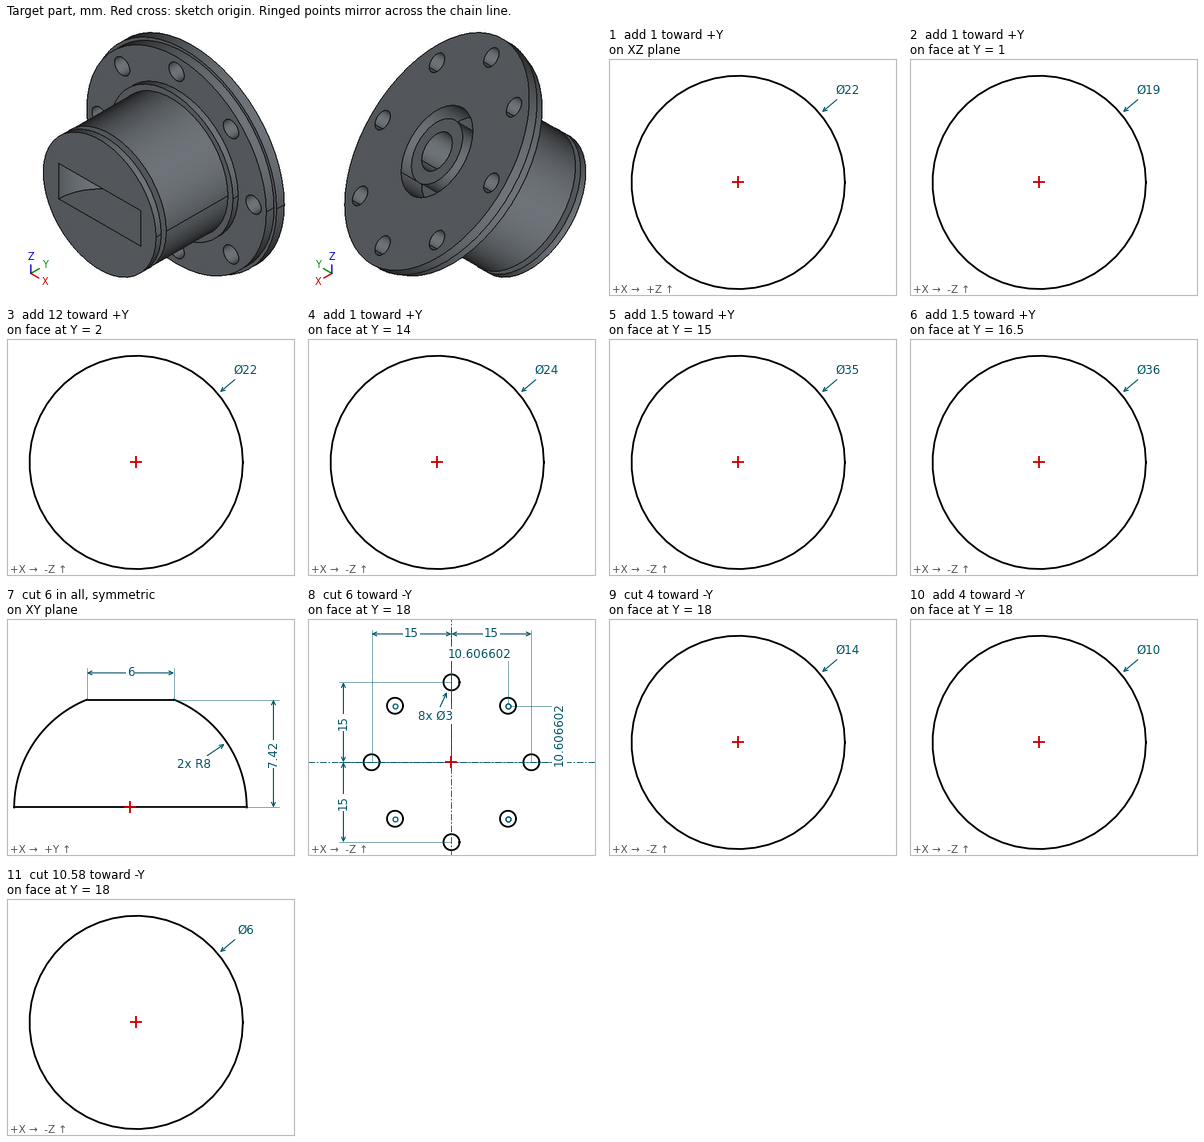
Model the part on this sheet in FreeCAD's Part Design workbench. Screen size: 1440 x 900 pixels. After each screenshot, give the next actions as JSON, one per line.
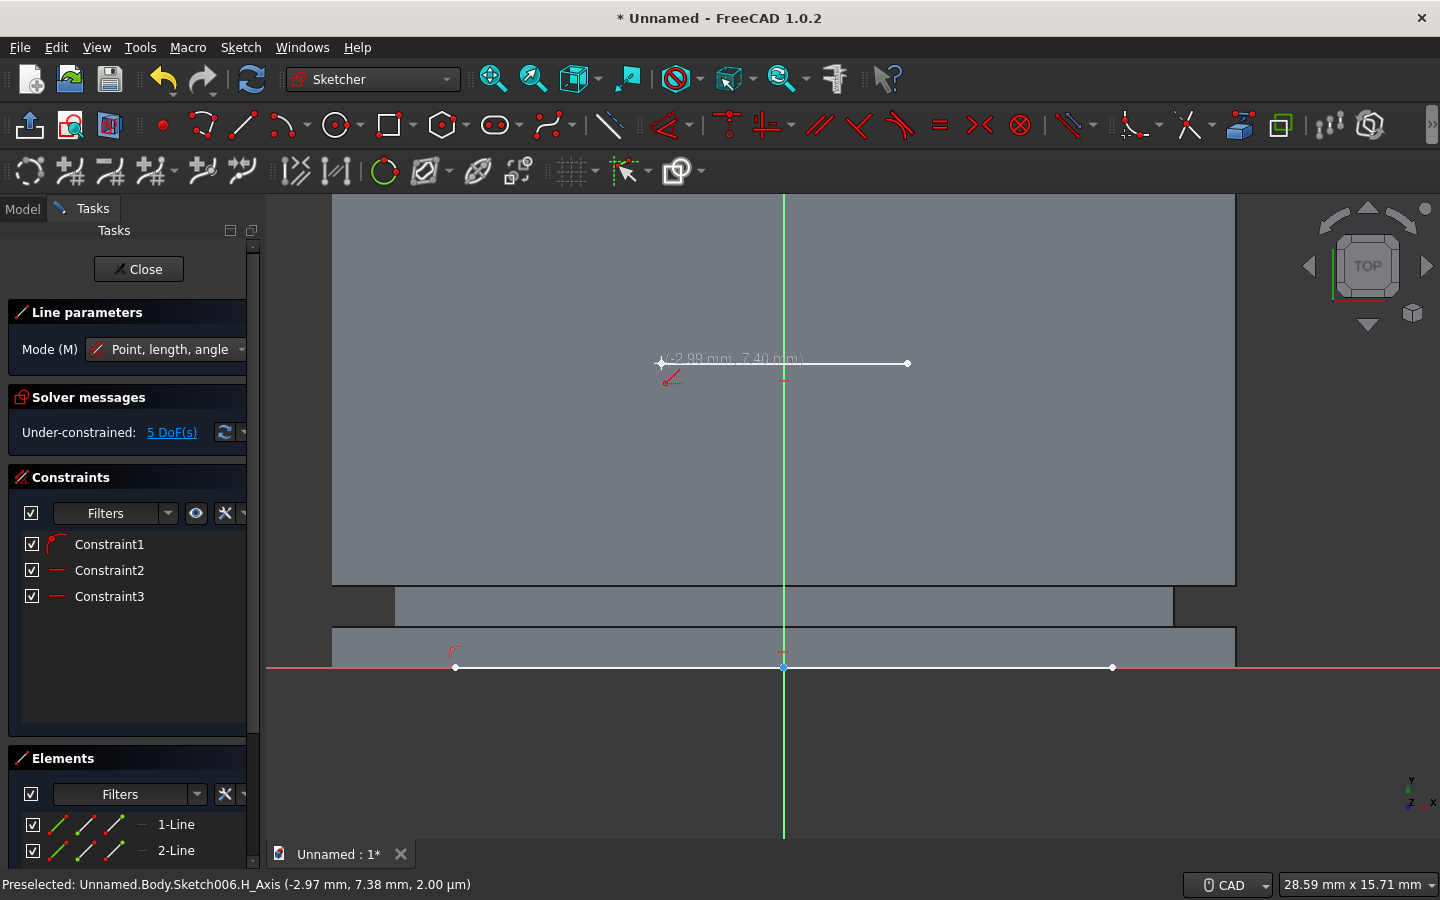
{"action": "left_click", "coordinate": [310, 126]}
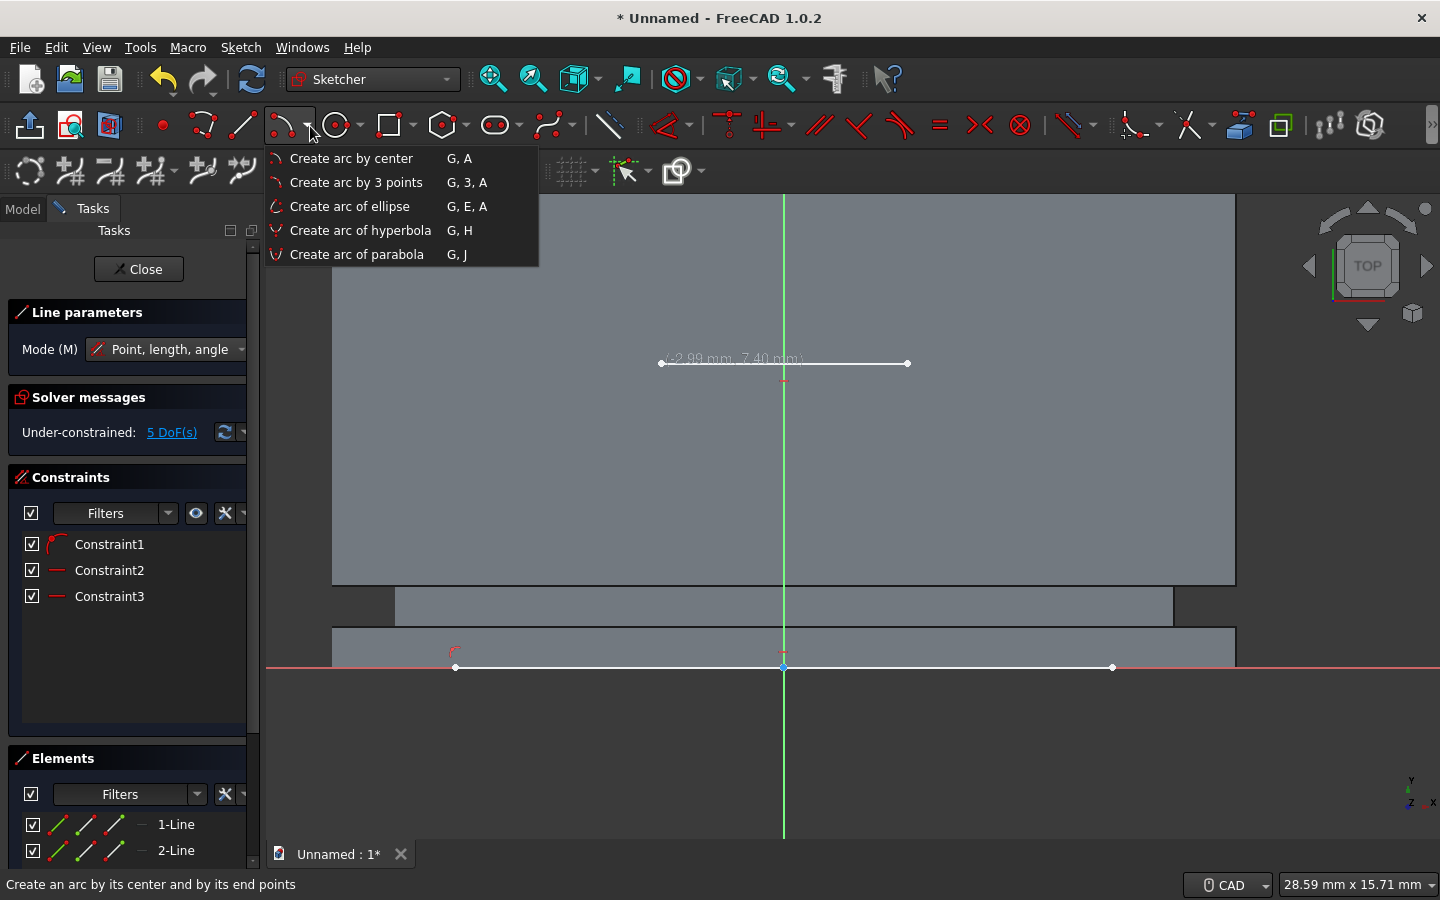
{"action": "left_click", "coordinate": [402, 182]}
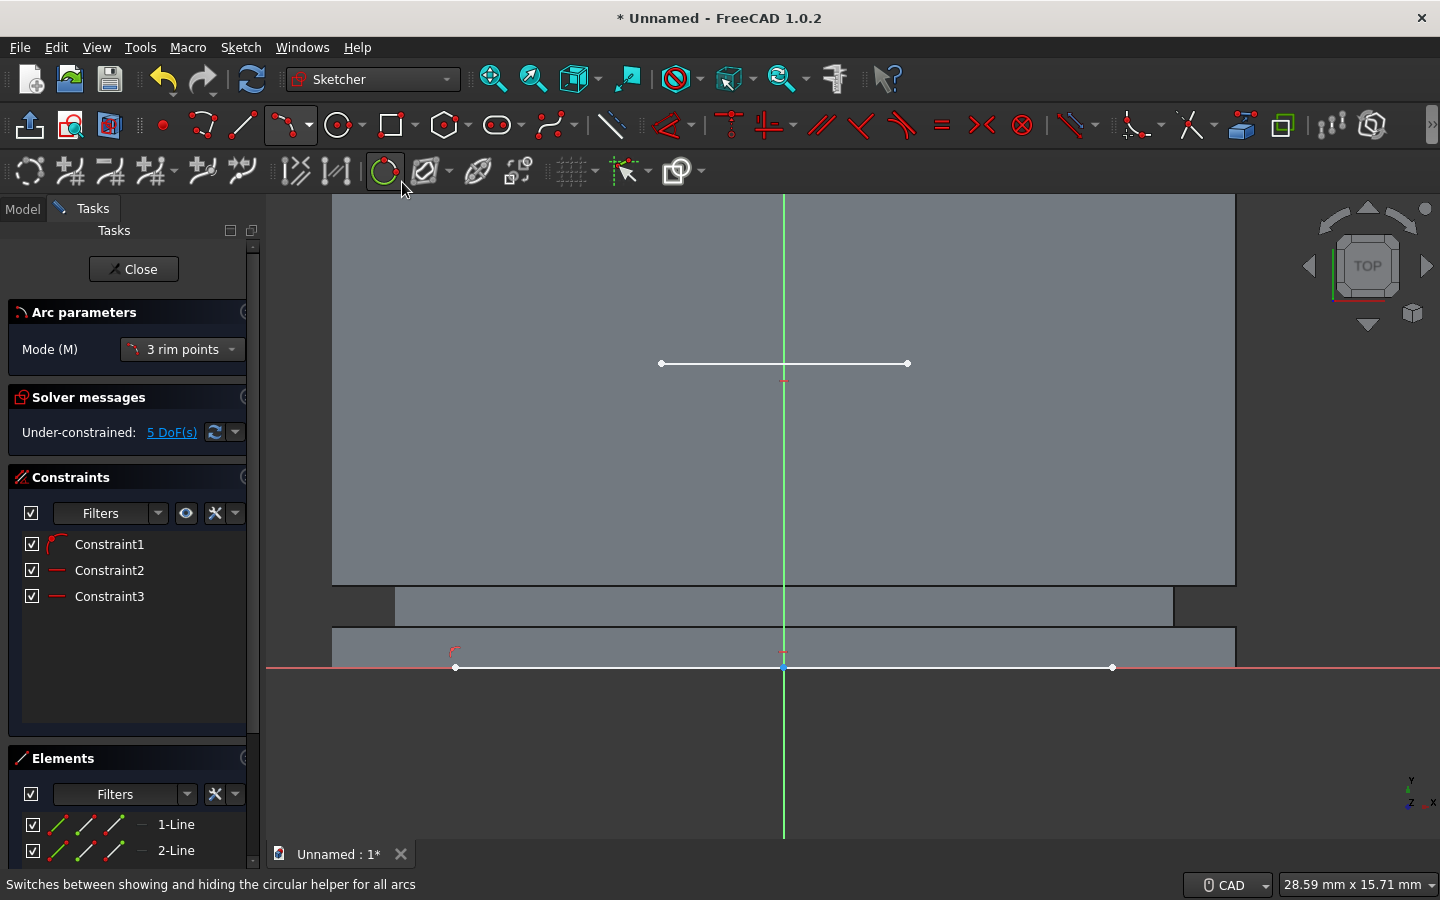
{"action": "left_click", "coordinate": [1112, 668]}
{"action": "left_click", "coordinate": [907, 364]}
{"action": "left_click", "coordinate": [1056, 484]}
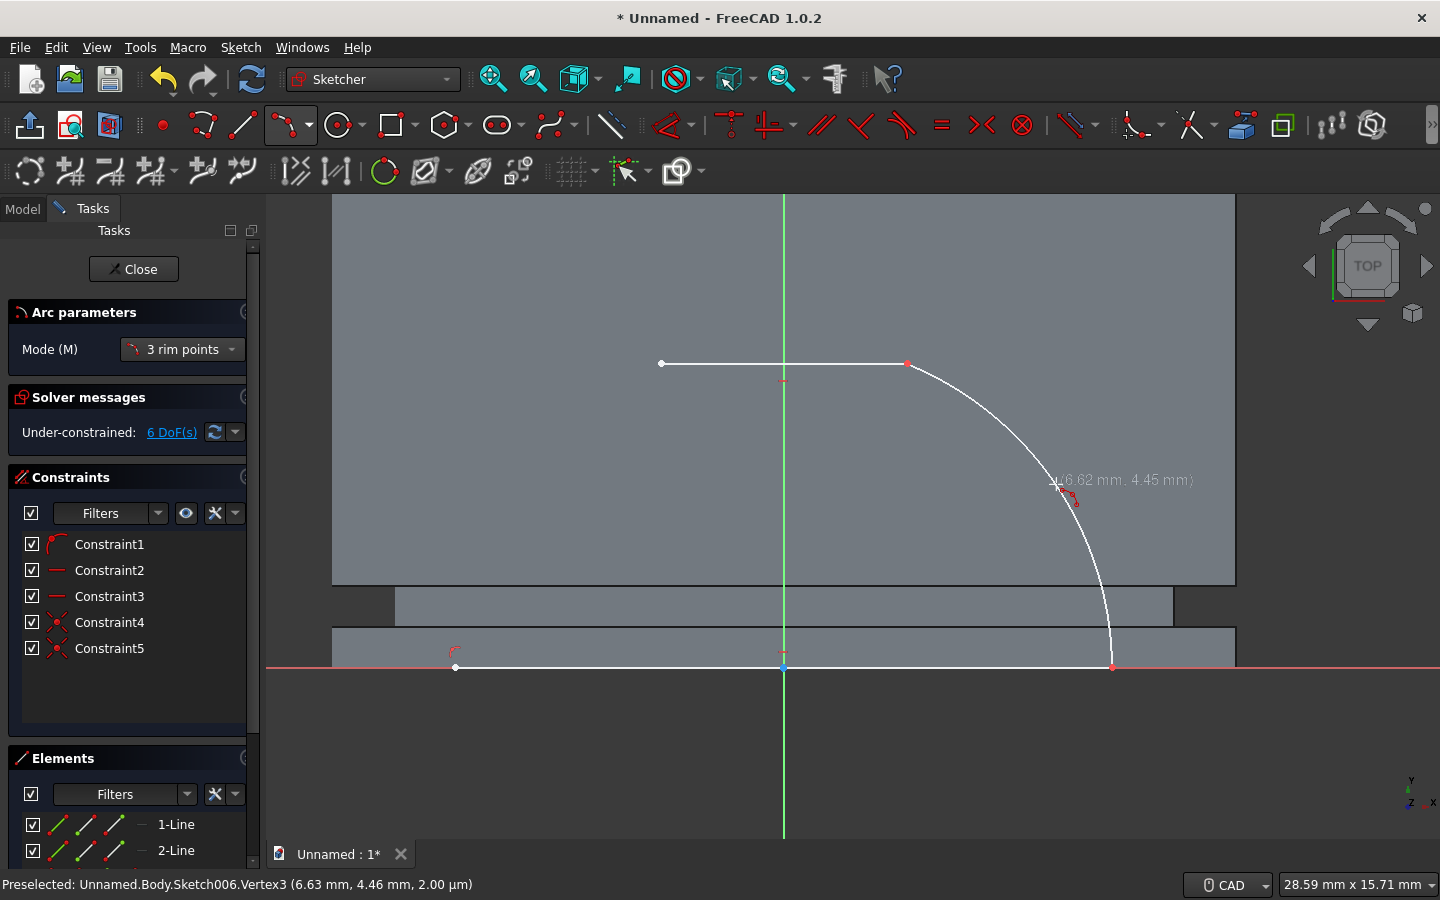
{"action": "left_click", "coordinate": [661, 364]}
{"action": "left_click", "coordinate": [455, 668]}
{"action": "left_click", "coordinate": [511, 484]}
{"action": "key", "text": "Escape"}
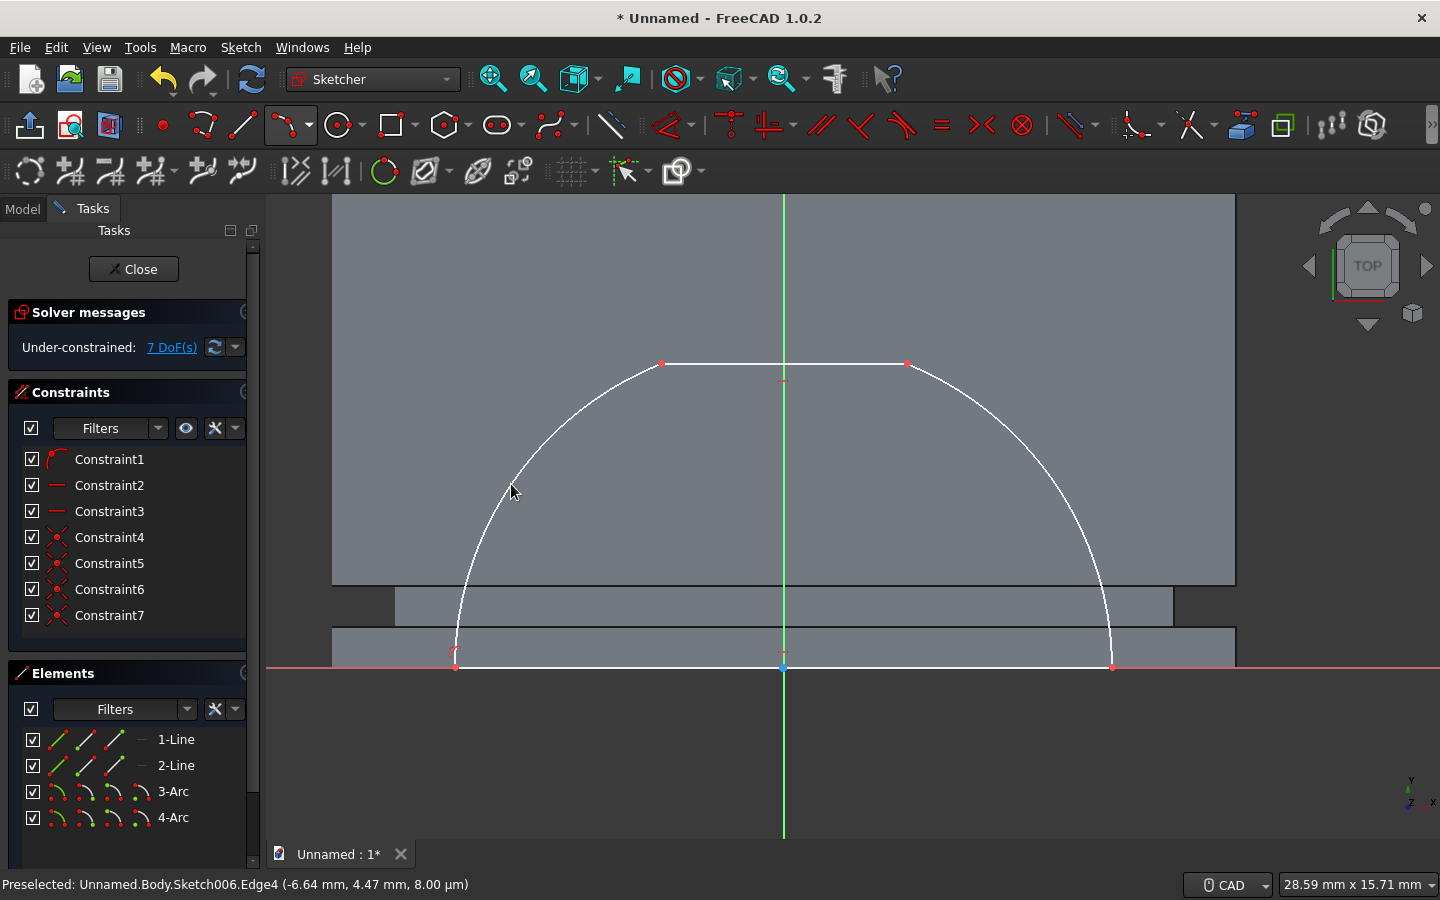
{"action": "left_click", "coordinate": [1091, 554]}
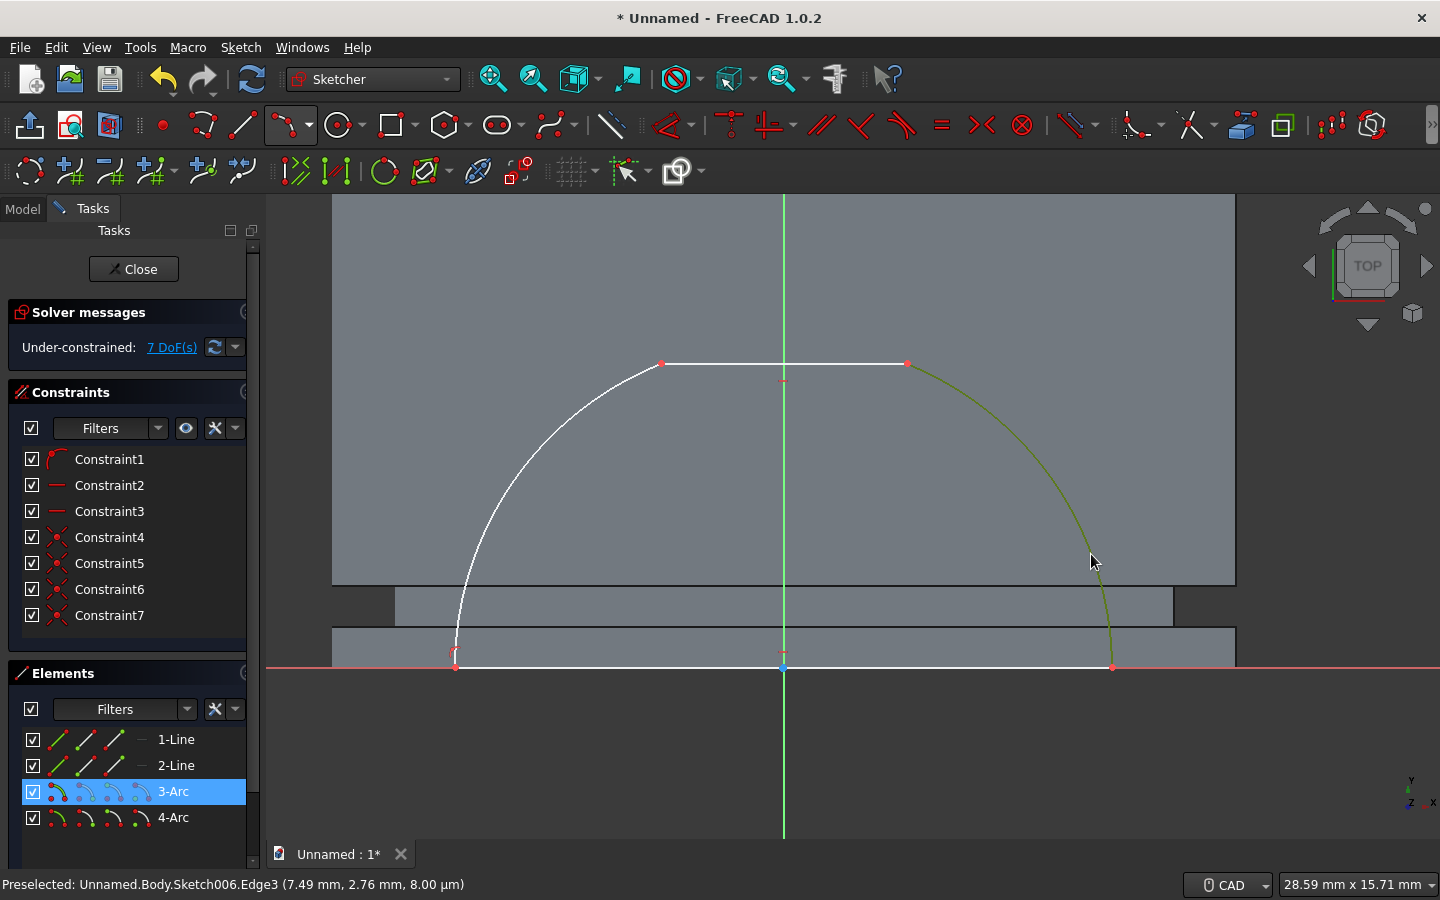
{"action": "left_click", "coordinate": [562, 426]}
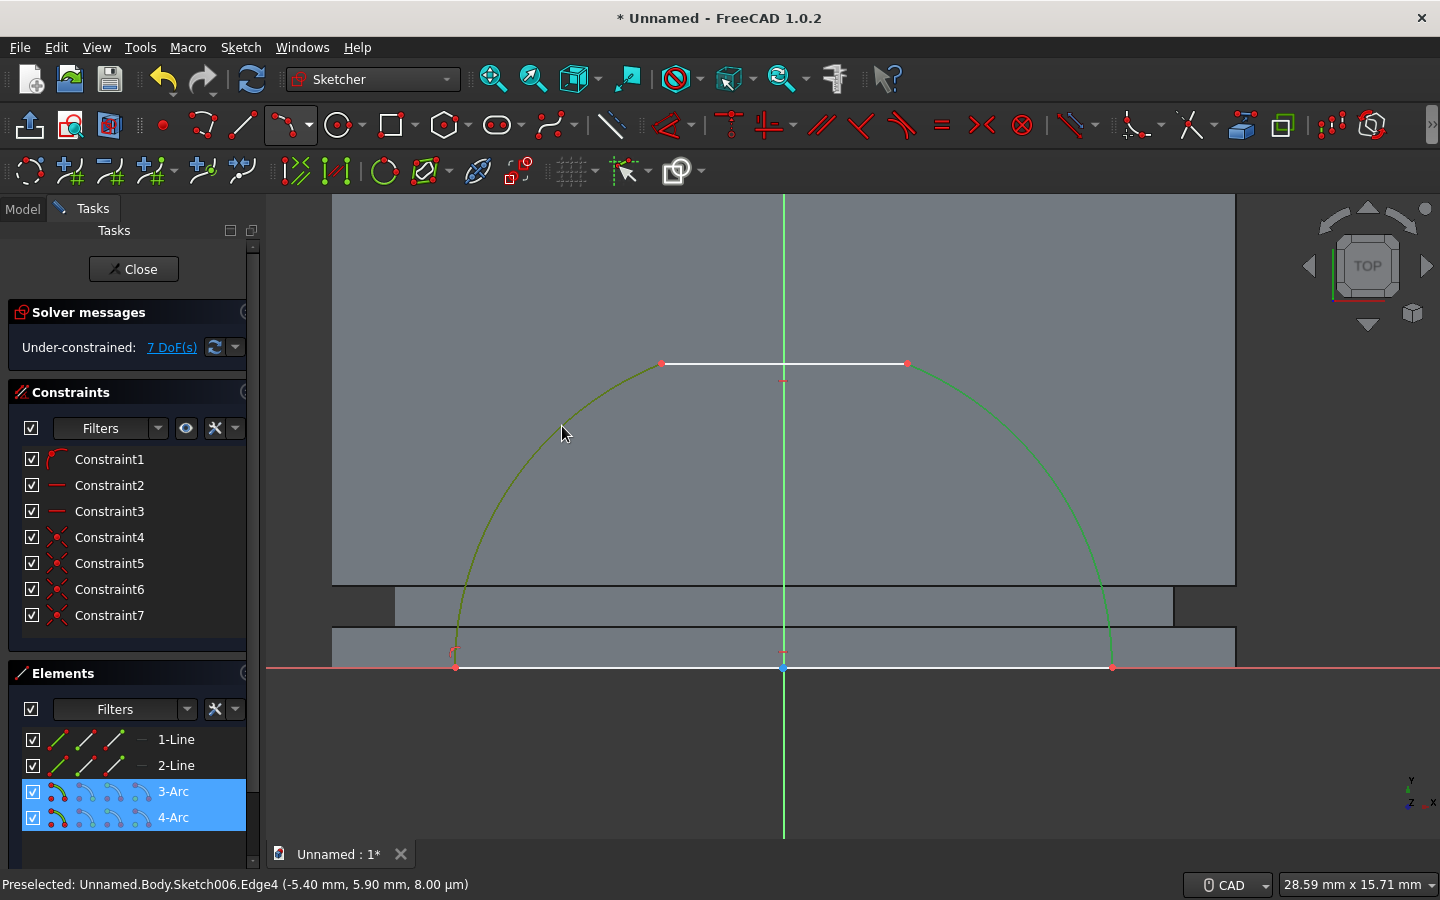
{"action": "left_click", "coordinate": [730, 126]}